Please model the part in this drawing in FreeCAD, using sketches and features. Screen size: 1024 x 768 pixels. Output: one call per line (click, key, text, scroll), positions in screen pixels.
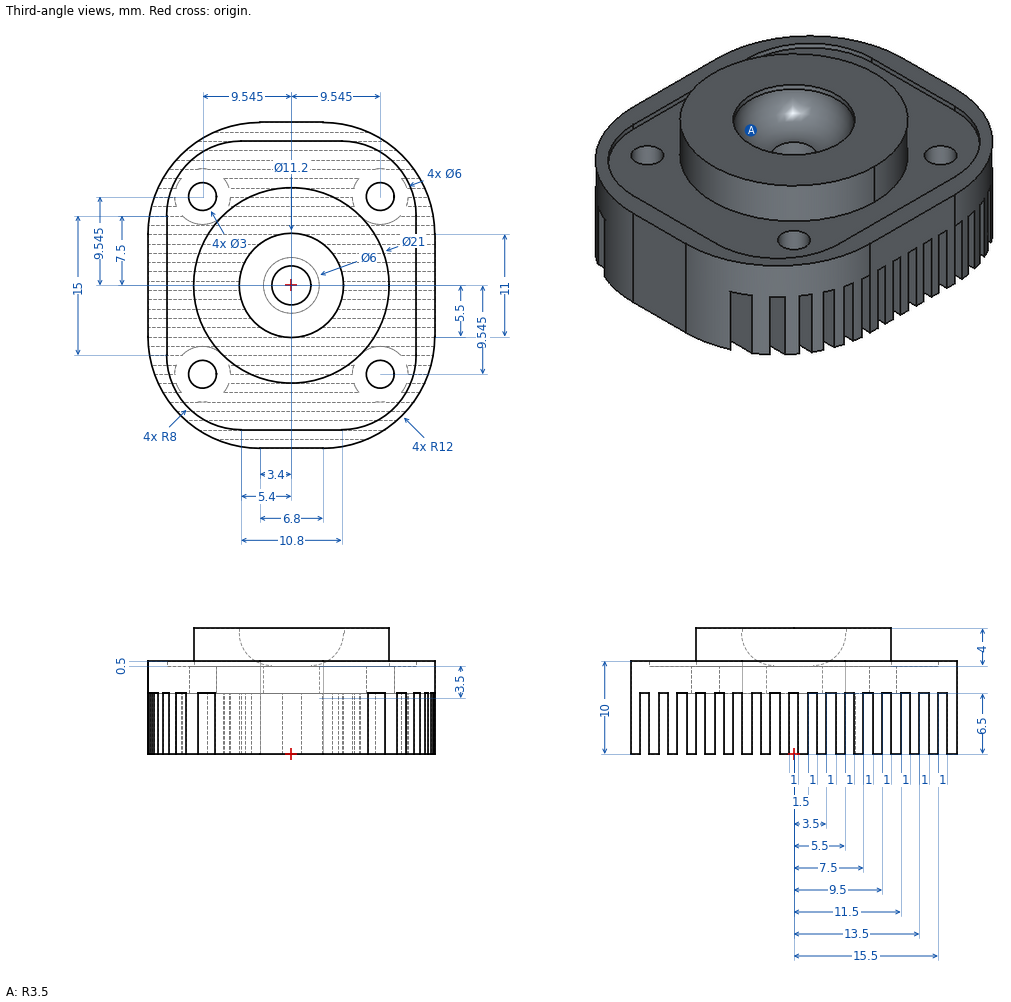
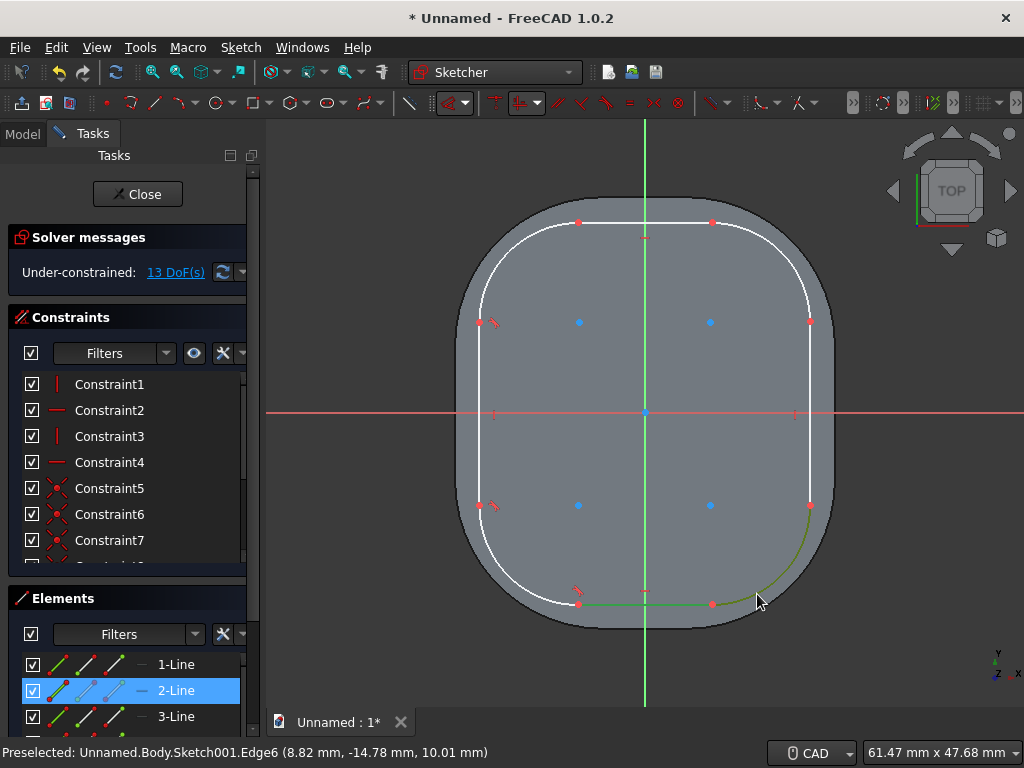
click(606, 104)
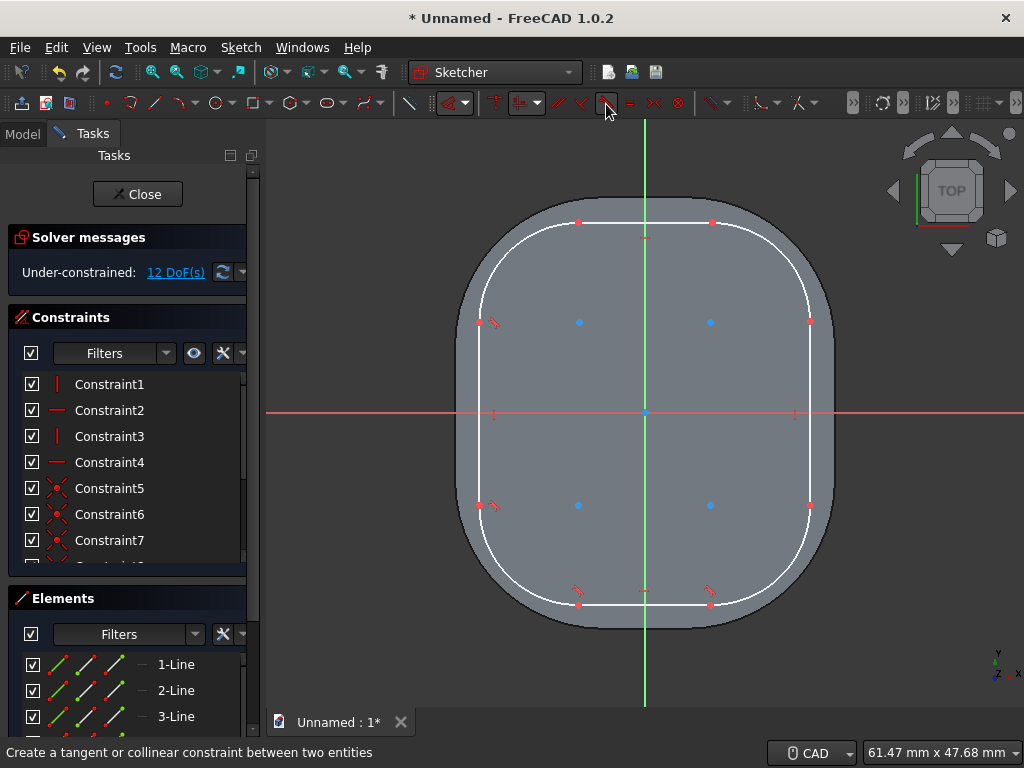
click(810, 451)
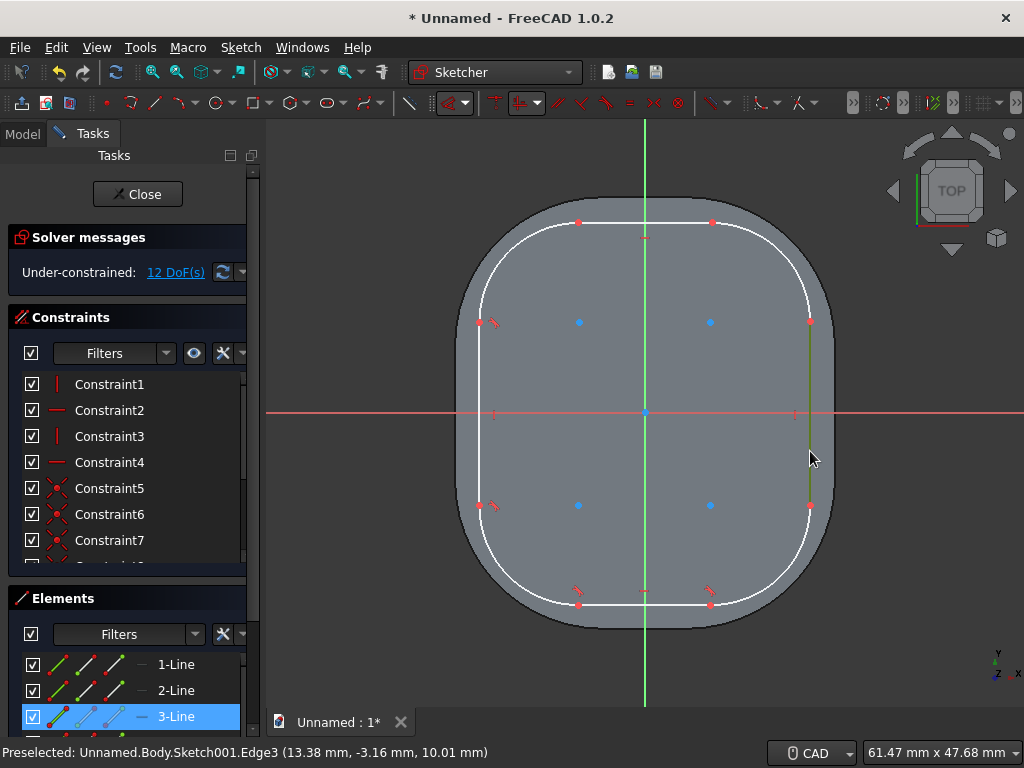
click(756, 594)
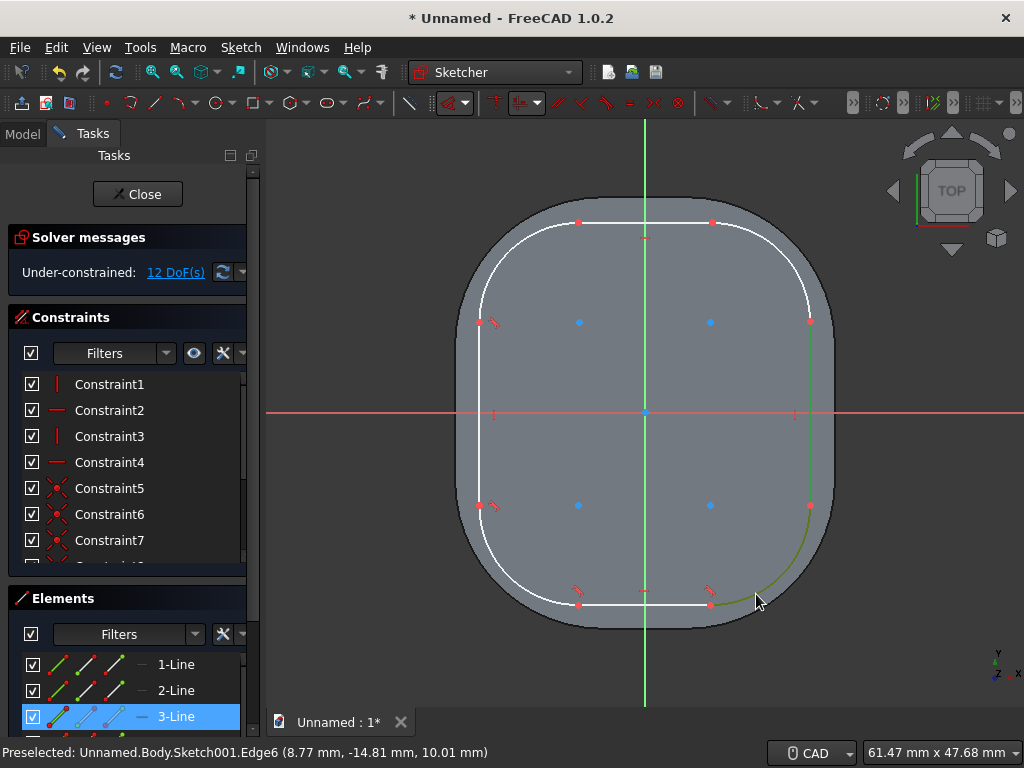
click(606, 104)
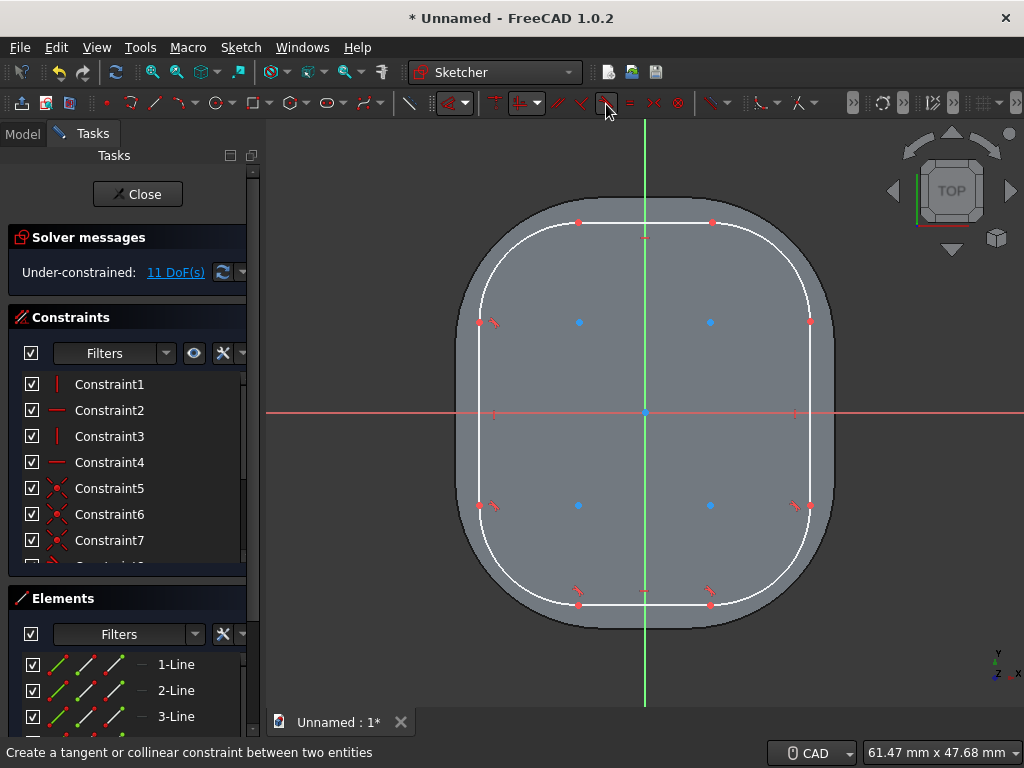
click(810, 451)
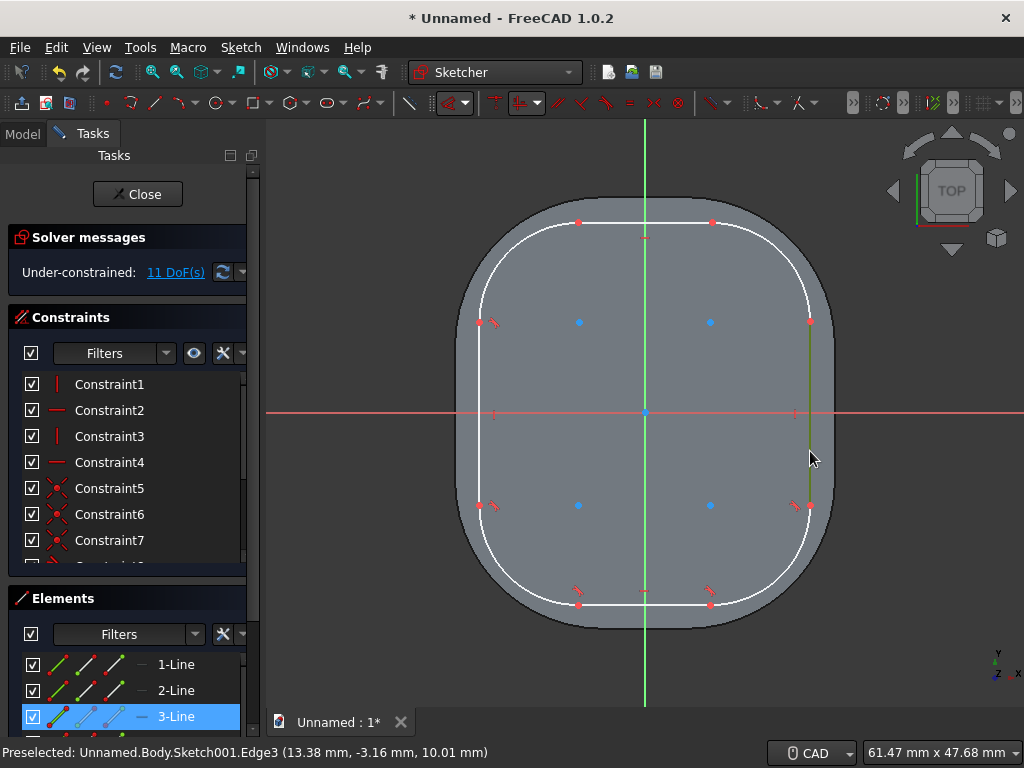
click(799, 277)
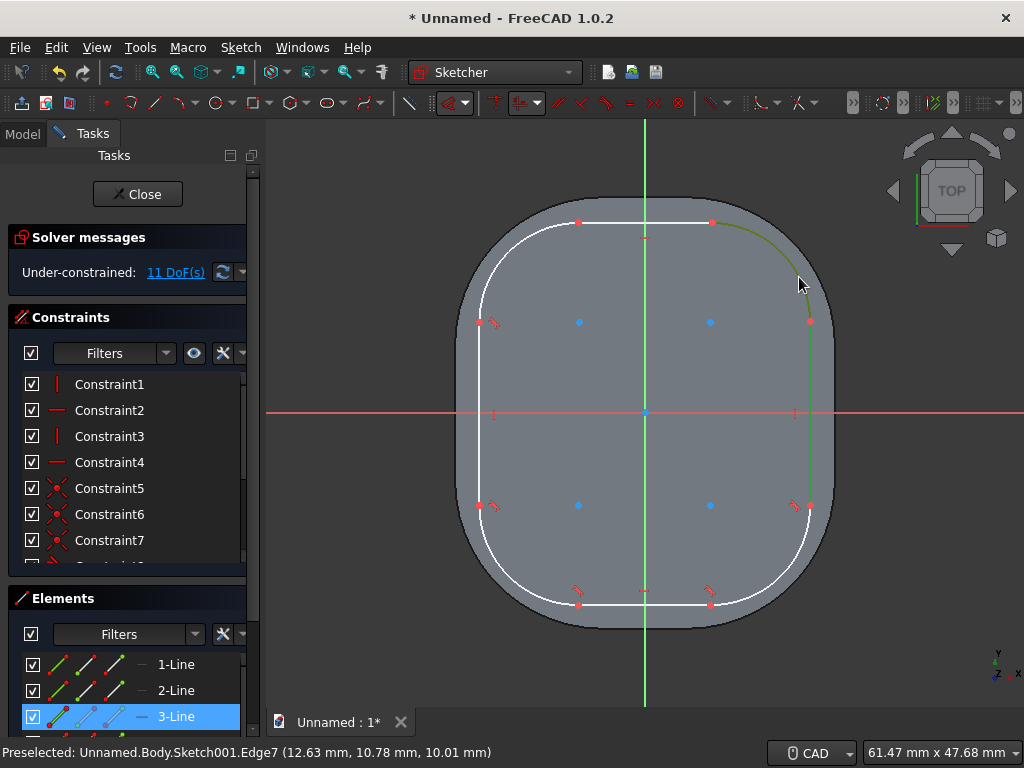
click(606, 104)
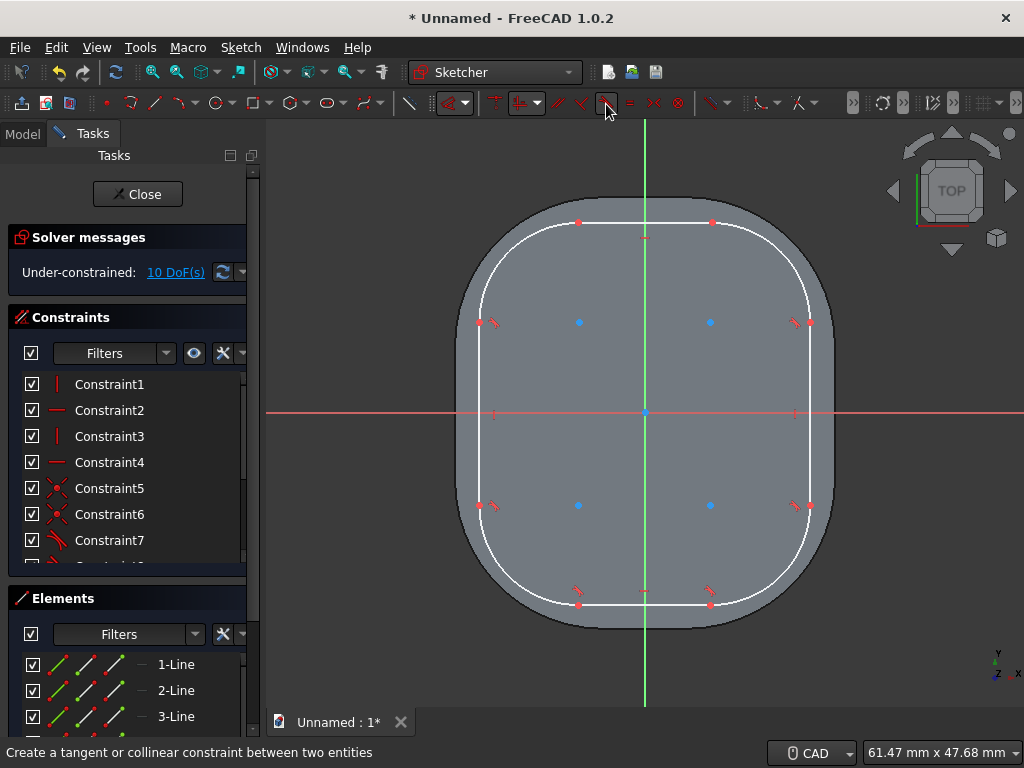
click(672, 223)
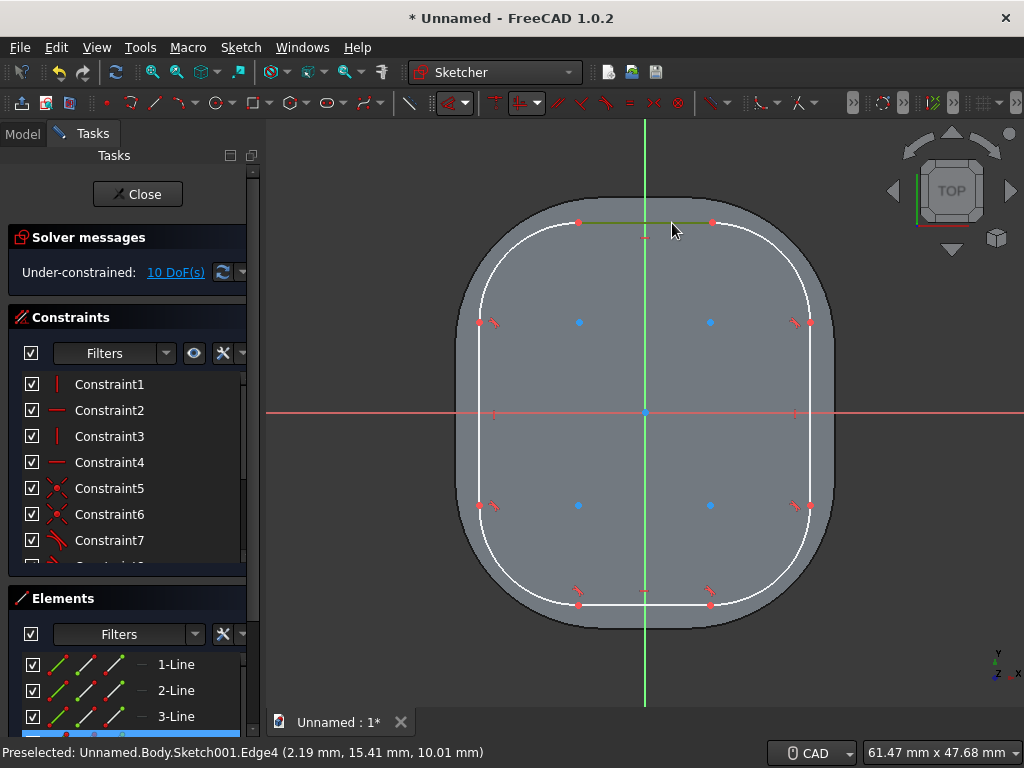
click(799, 277)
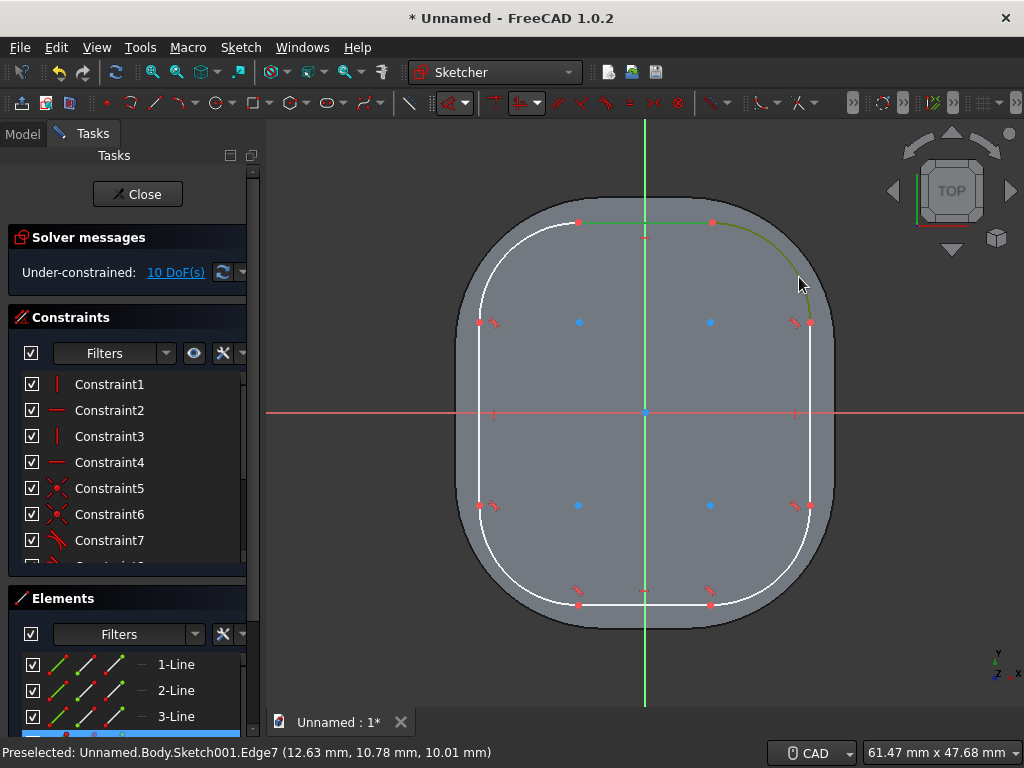
key(t)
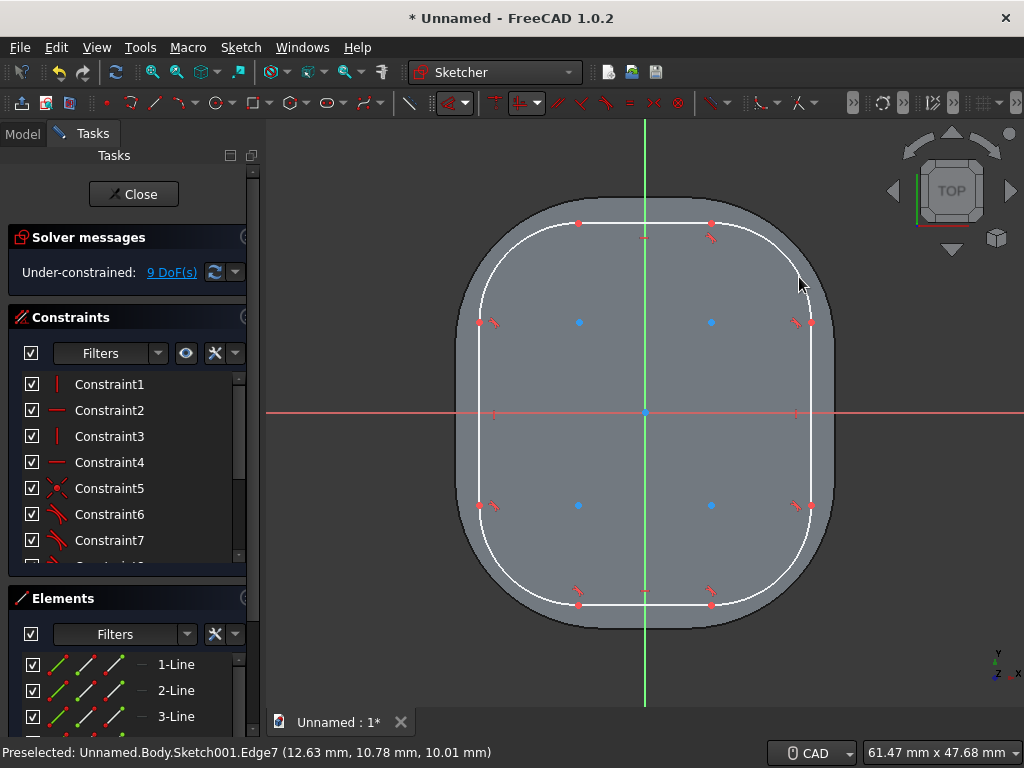
click(672, 223)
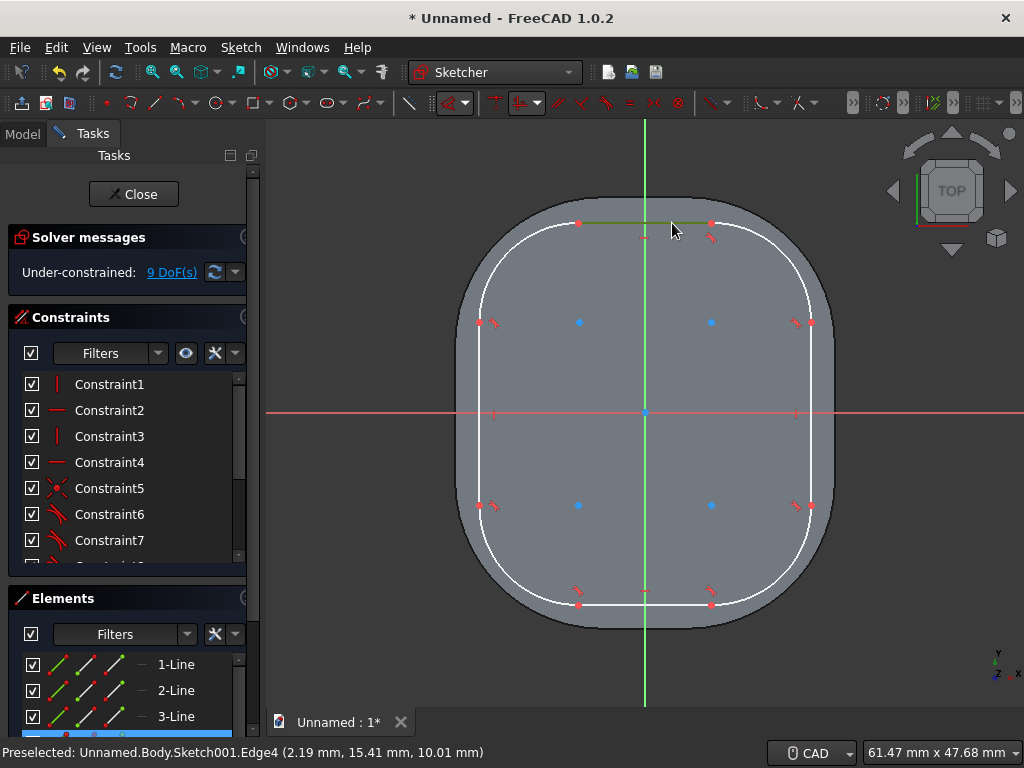
click(533, 234)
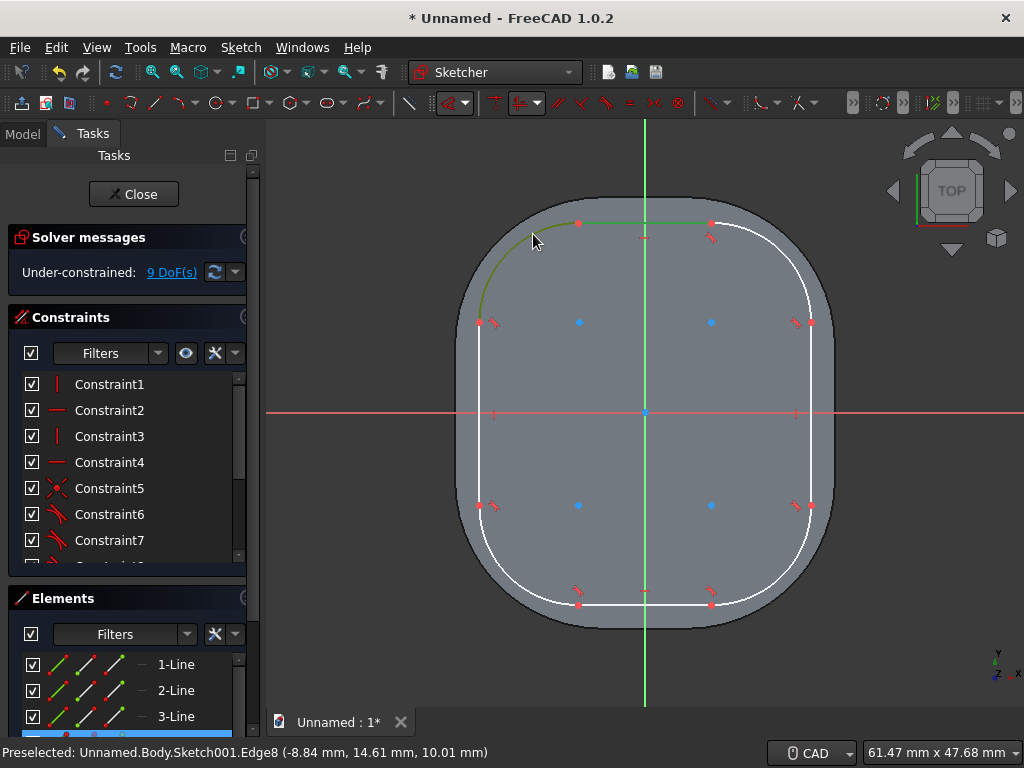
click(606, 104)